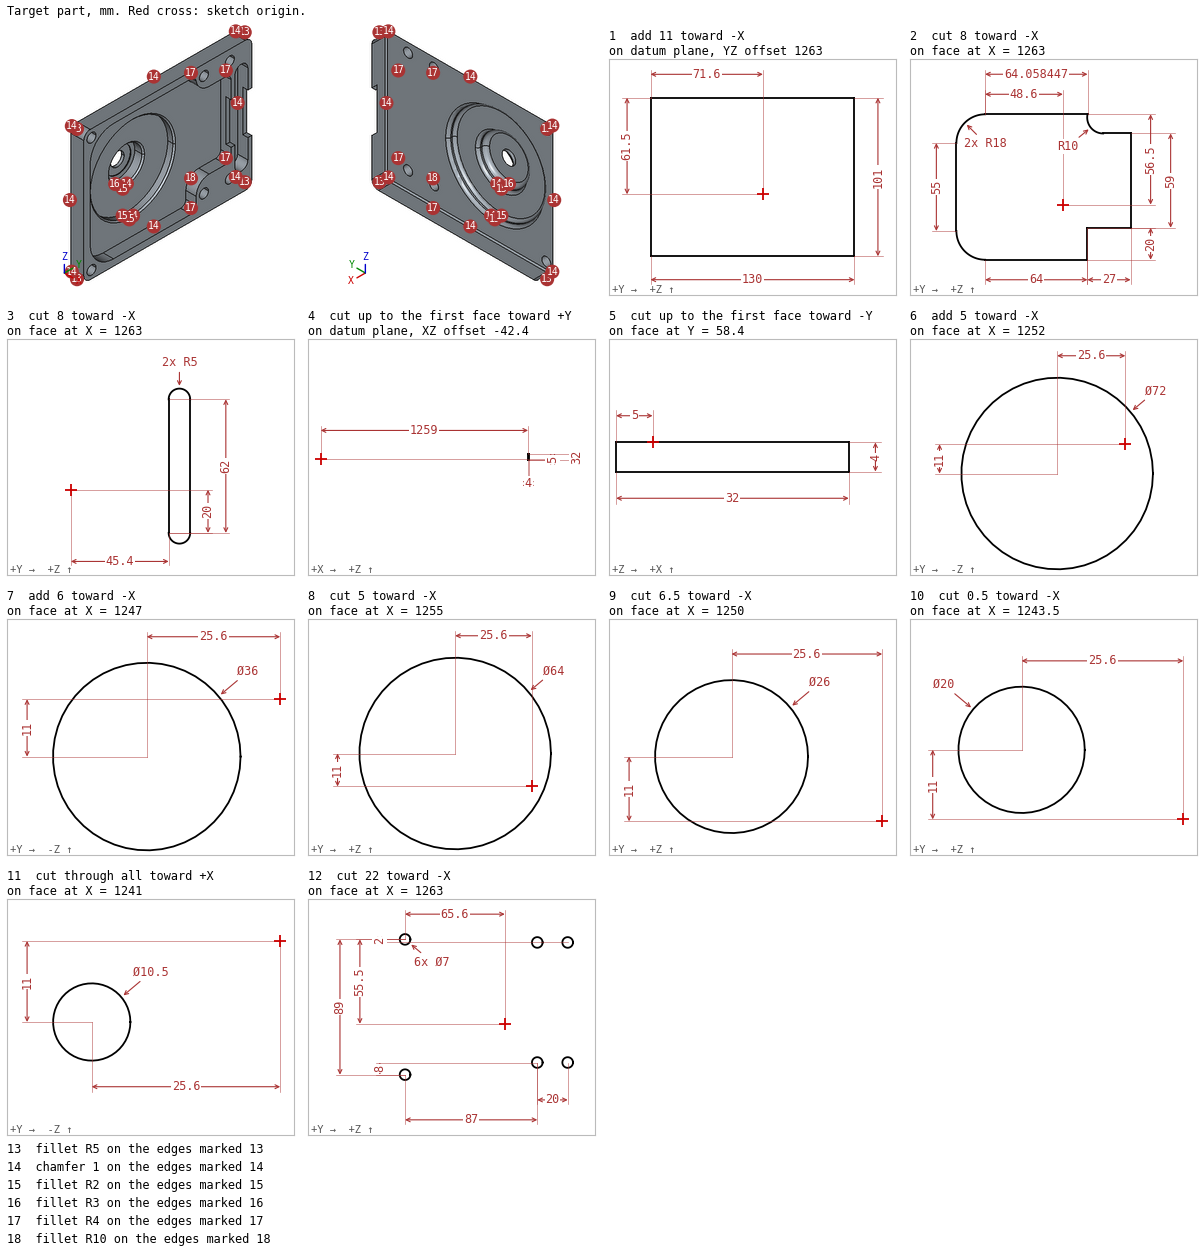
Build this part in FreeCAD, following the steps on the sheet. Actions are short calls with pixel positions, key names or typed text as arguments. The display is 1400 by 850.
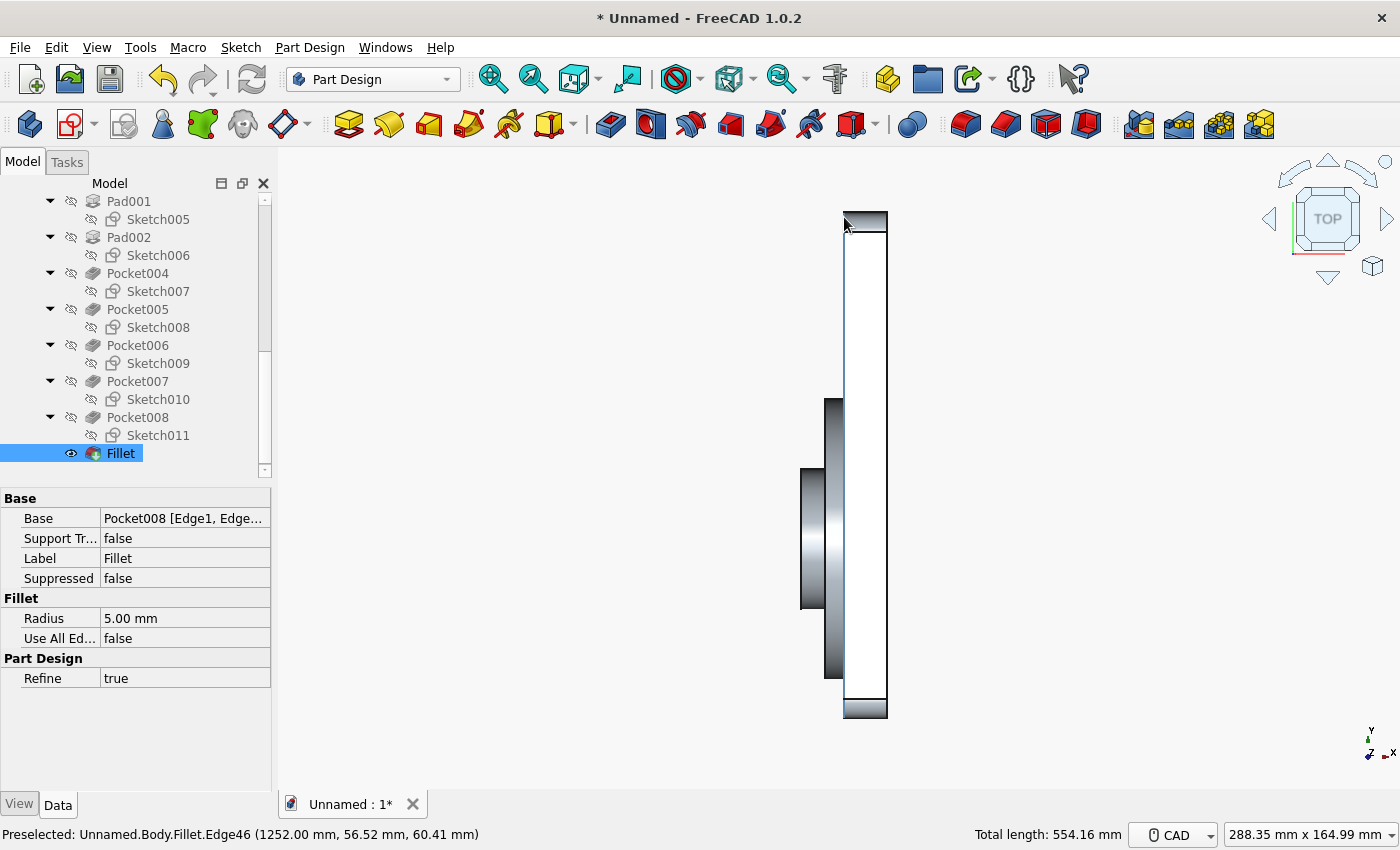
key(1)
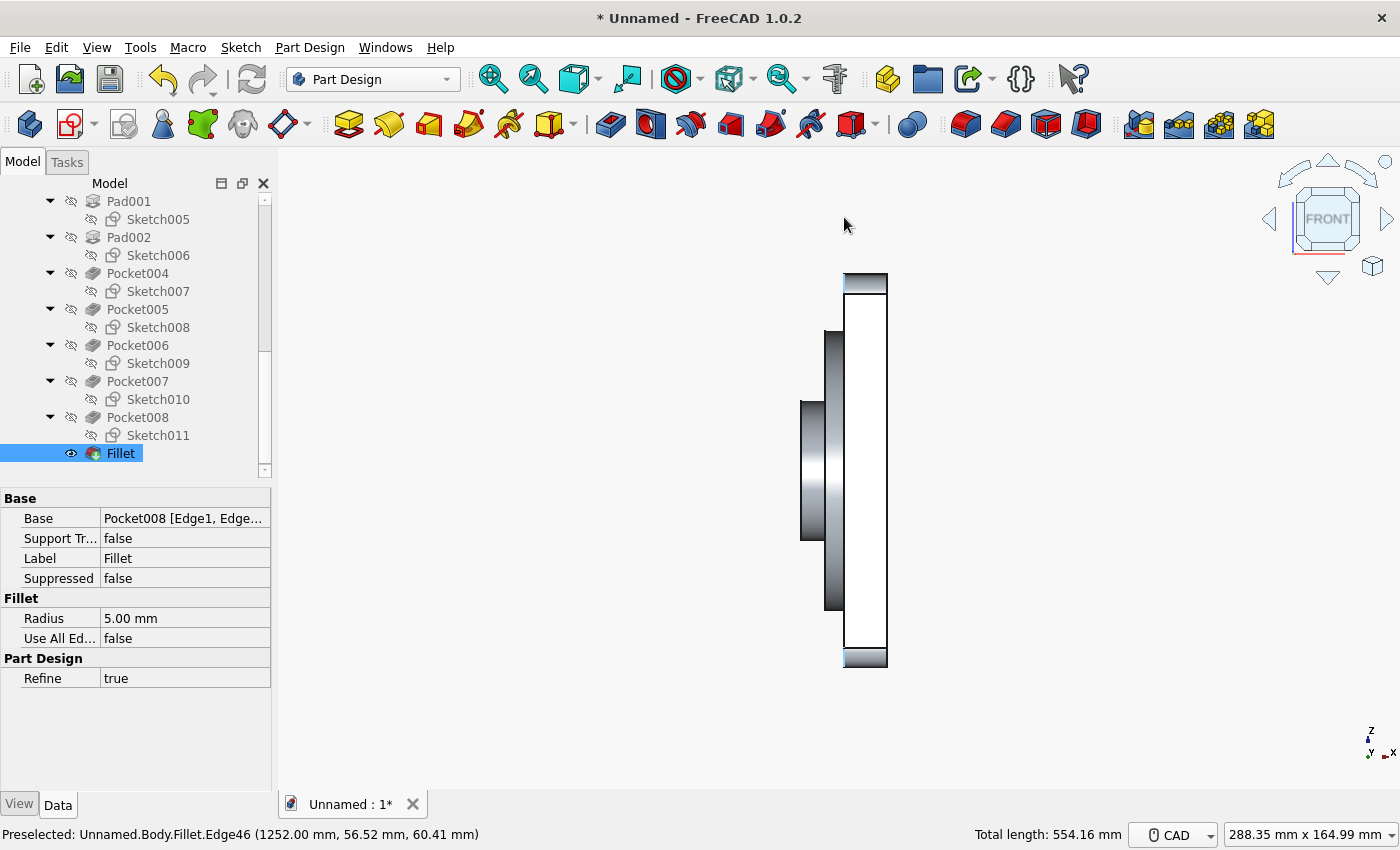
click(844, 470, ctrl)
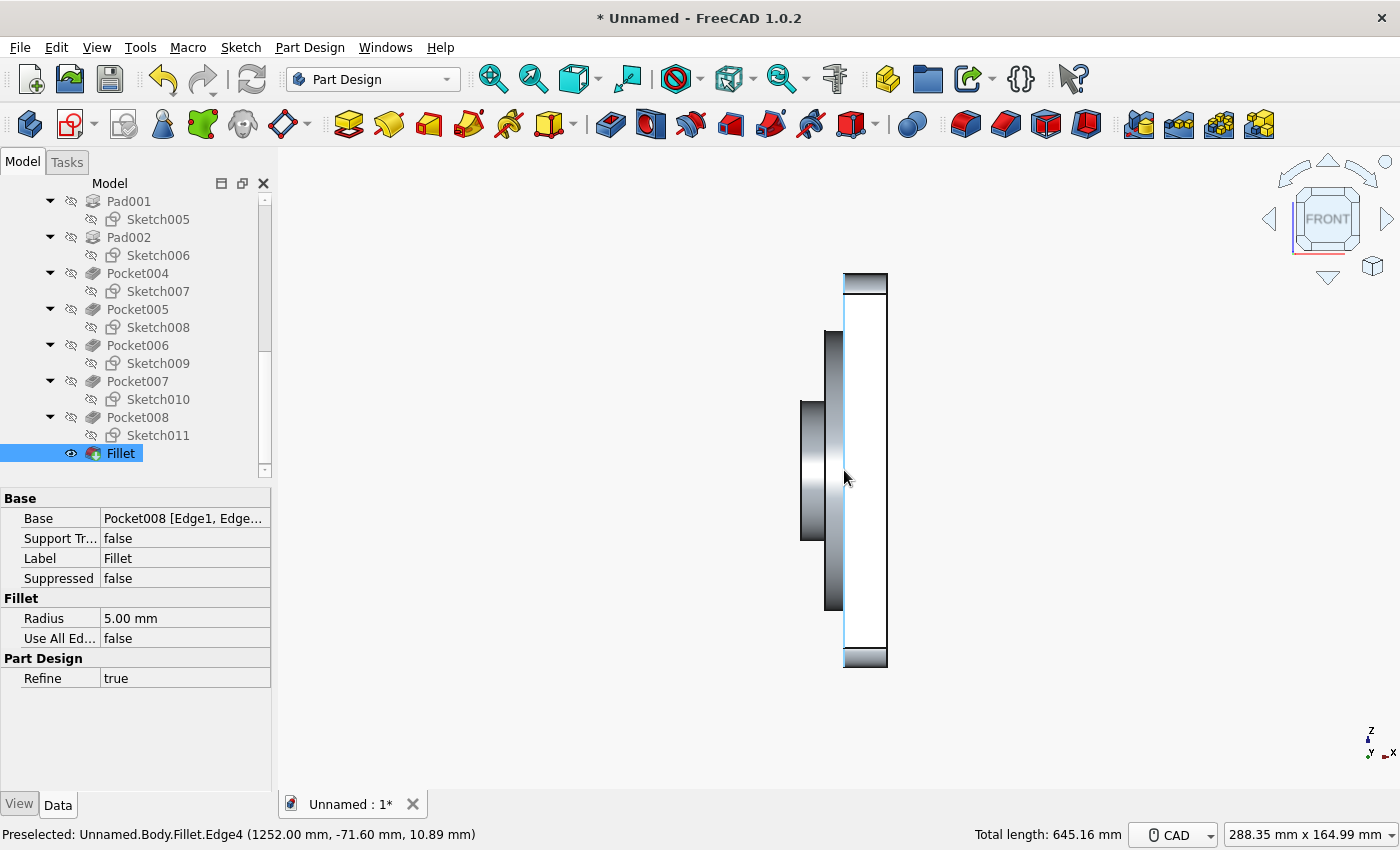
key(3)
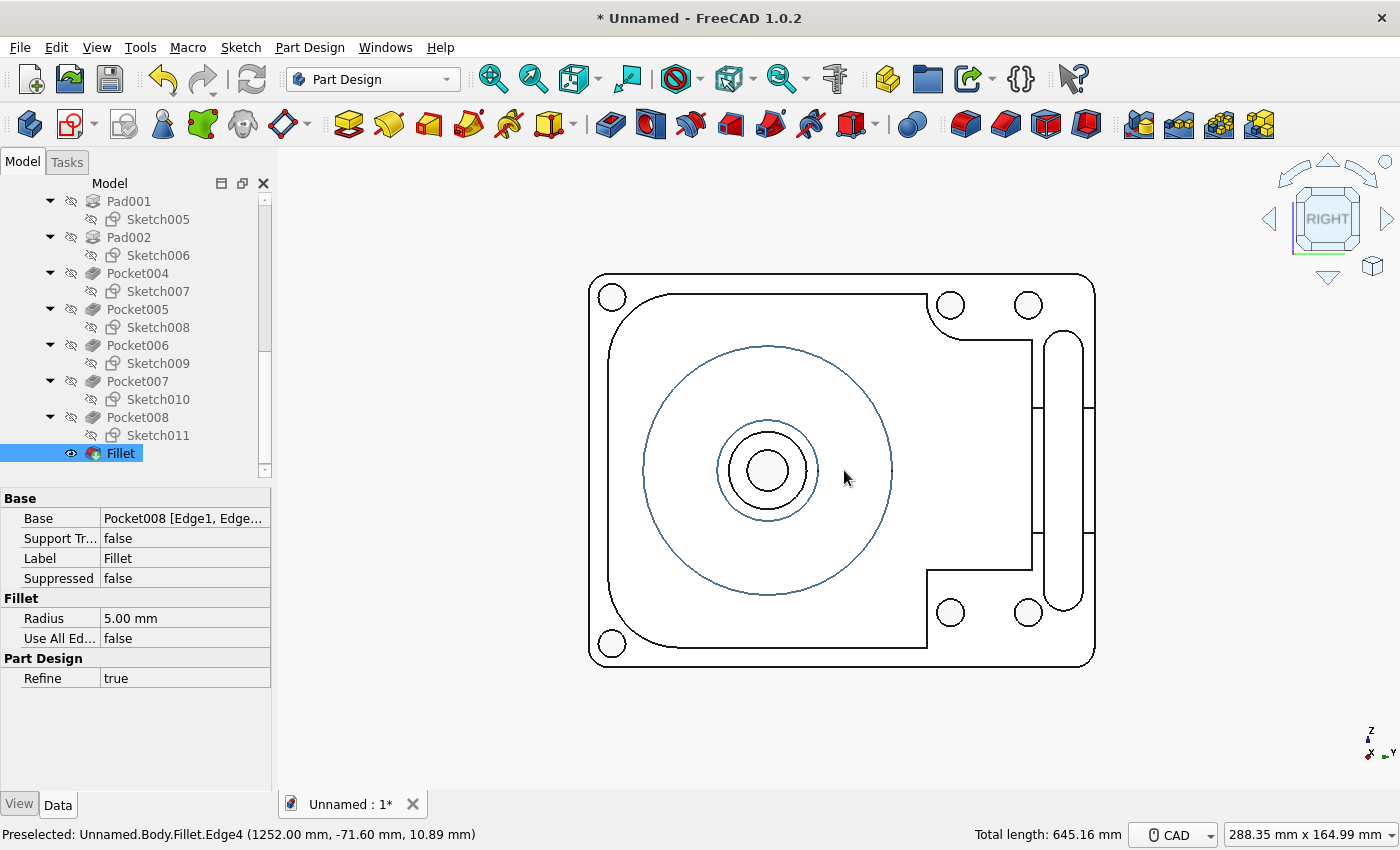
key(5)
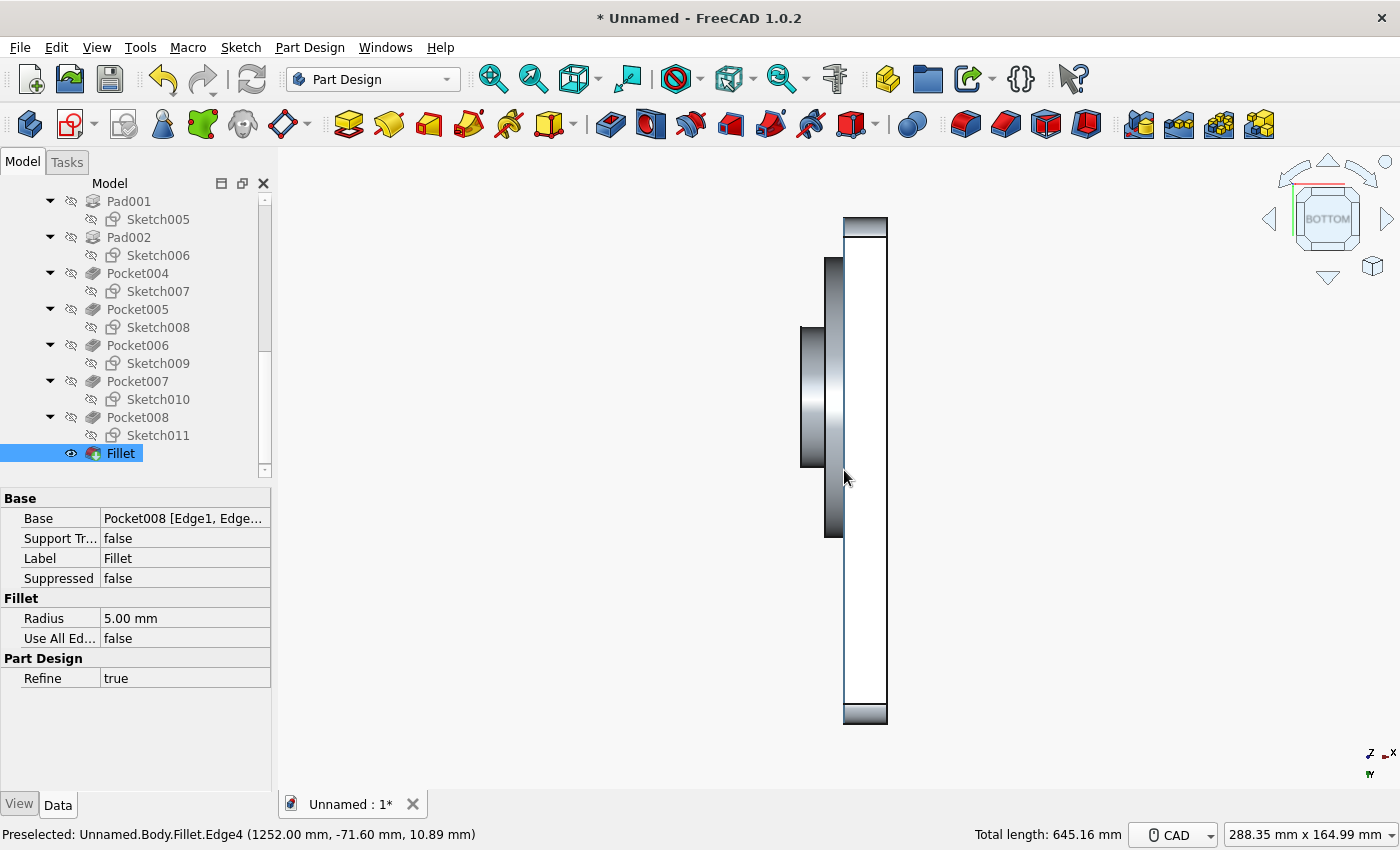
key(4)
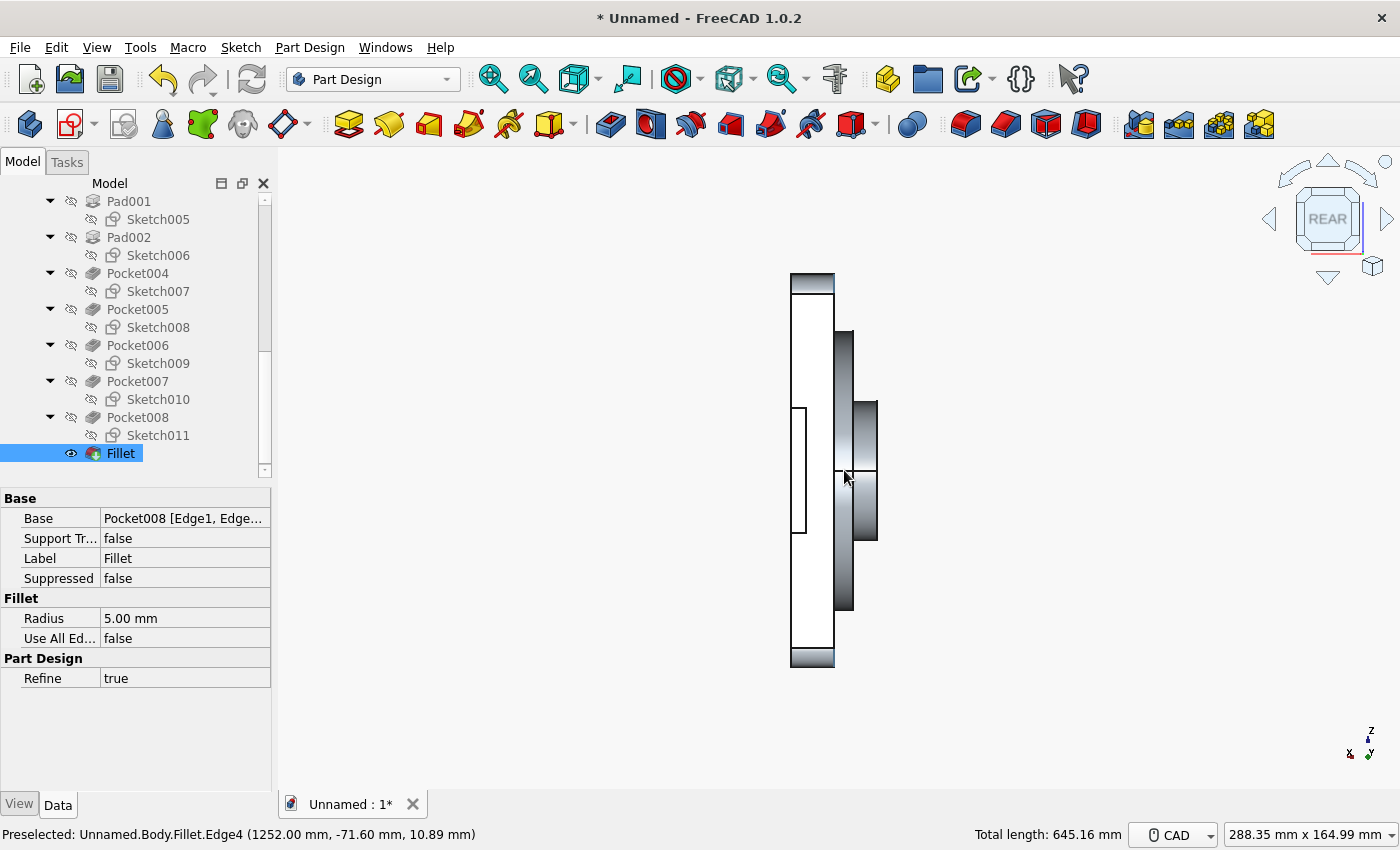
click(834, 470, ctrl)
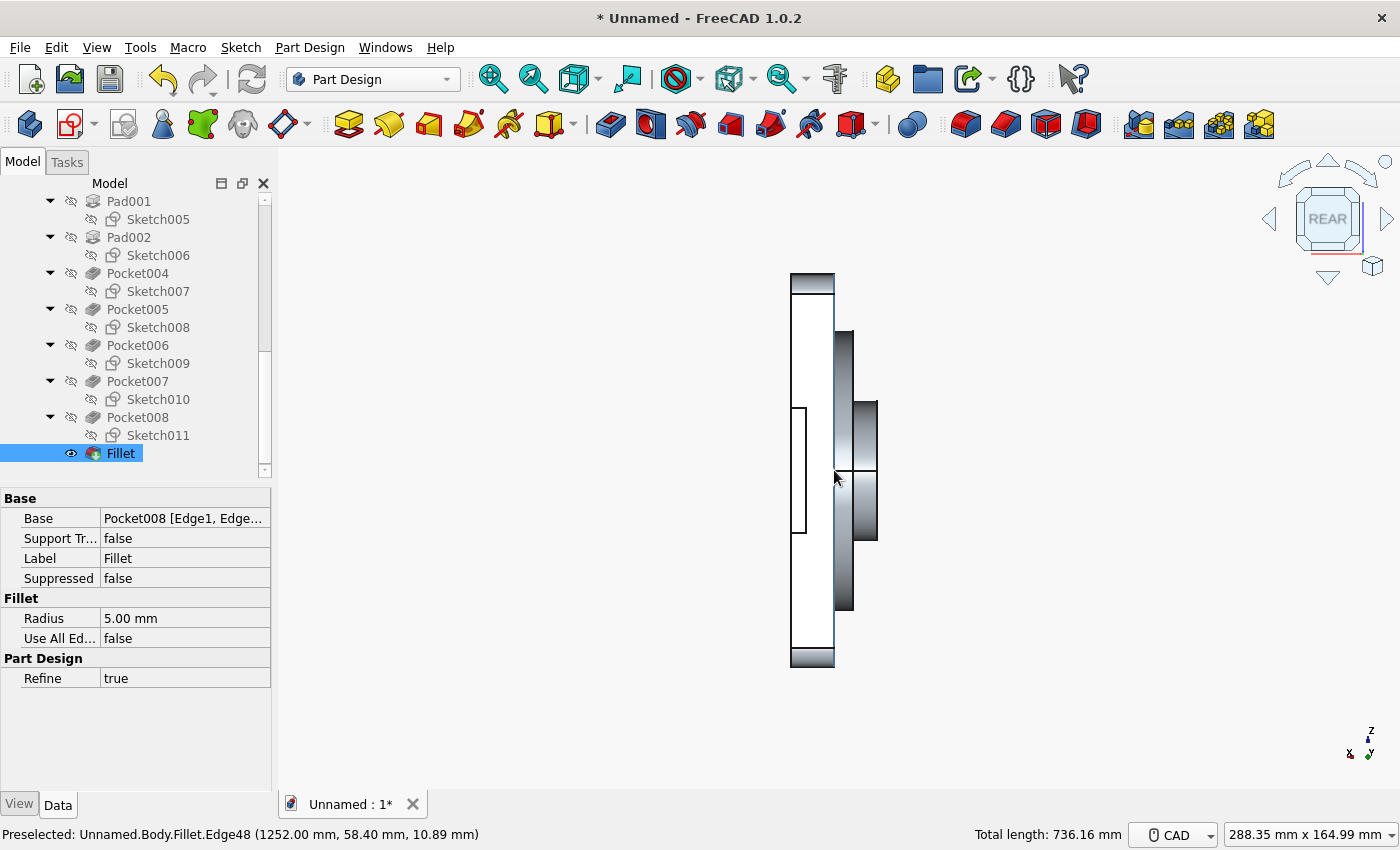
click(1006, 124)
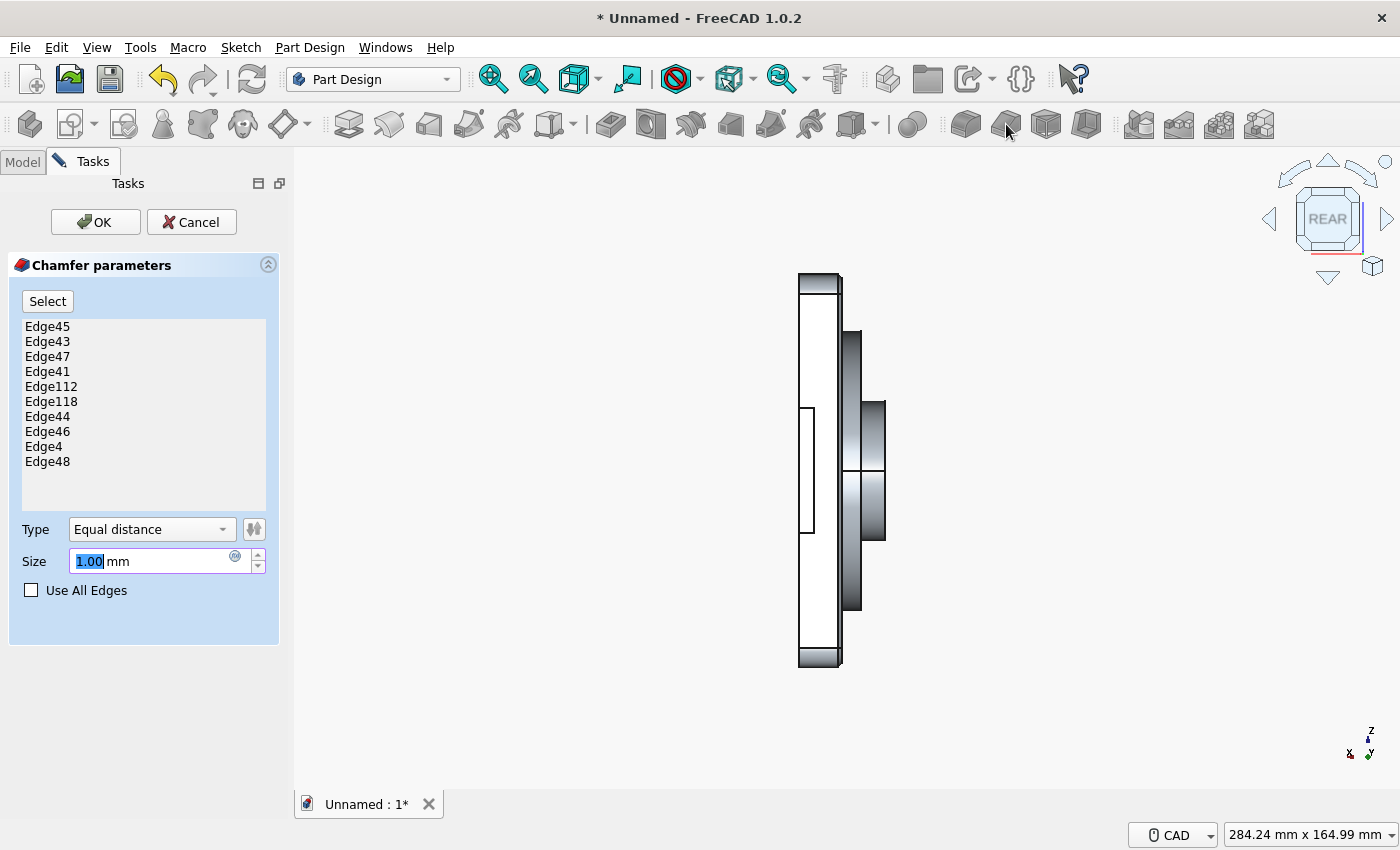
text(1)
key(Tab)